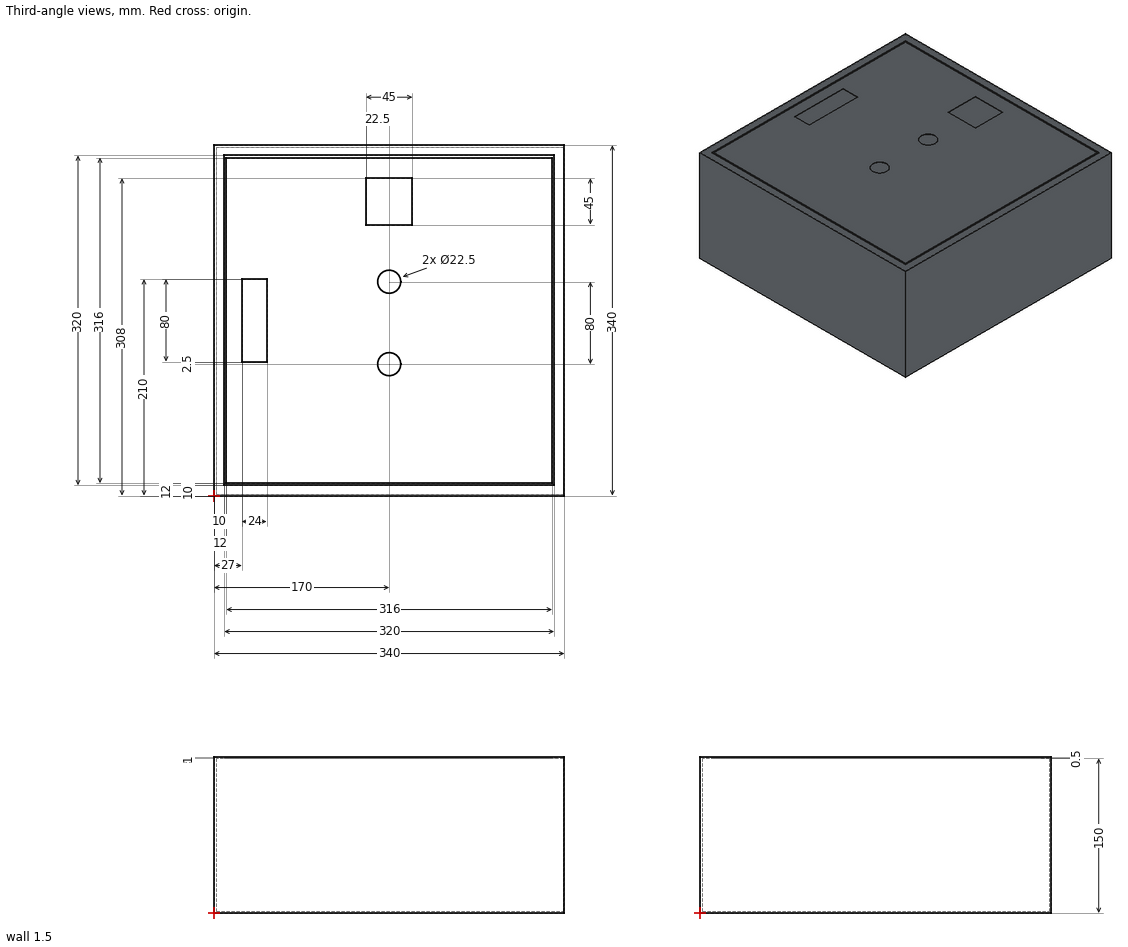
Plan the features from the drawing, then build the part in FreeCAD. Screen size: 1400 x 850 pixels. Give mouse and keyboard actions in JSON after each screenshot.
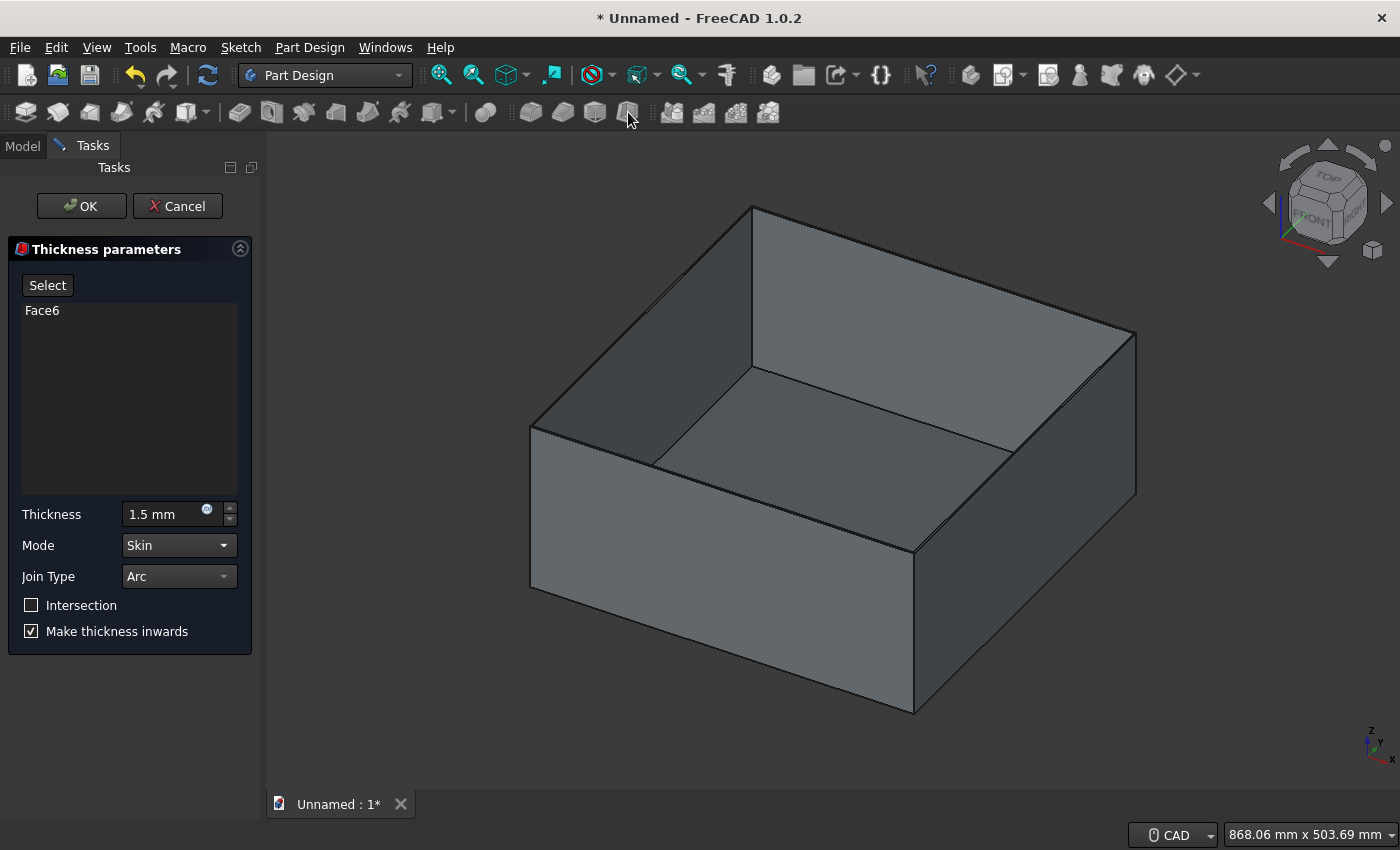
{"action": "left_click", "coordinate": [180, 576]}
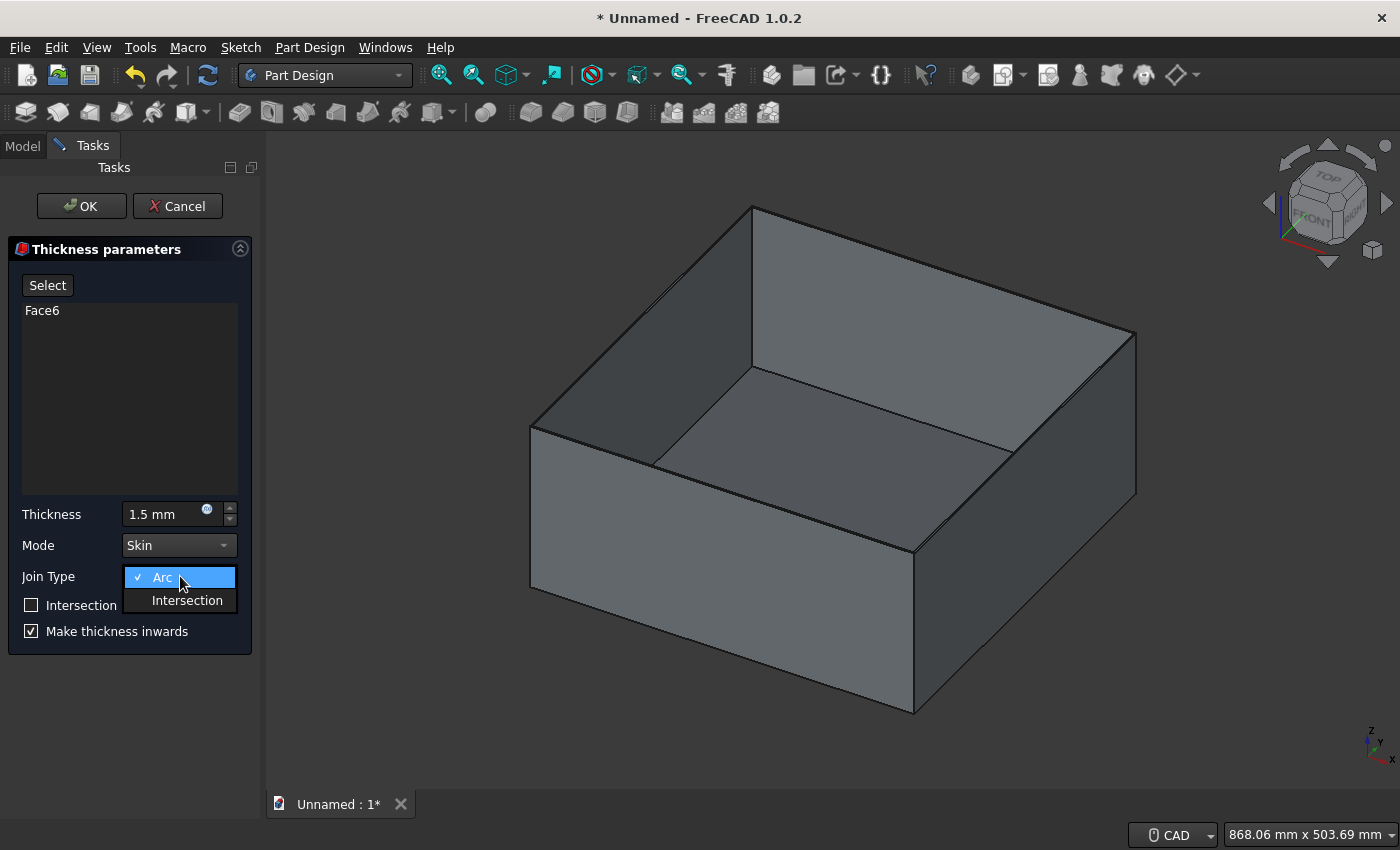
{"action": "left_click", "coordinate": [179, 600]}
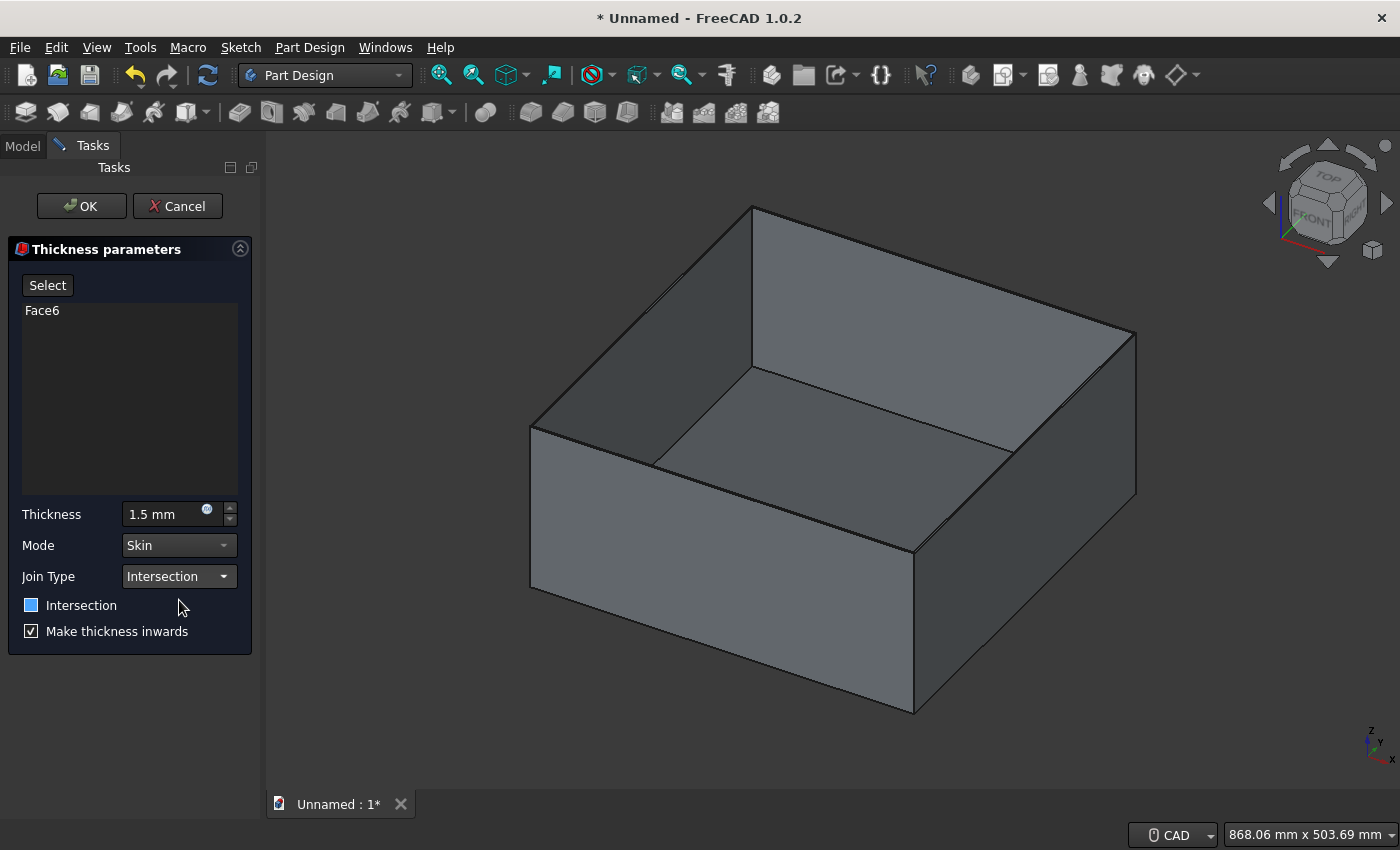
{"action": "left_click", "coordinate": [82, 206]}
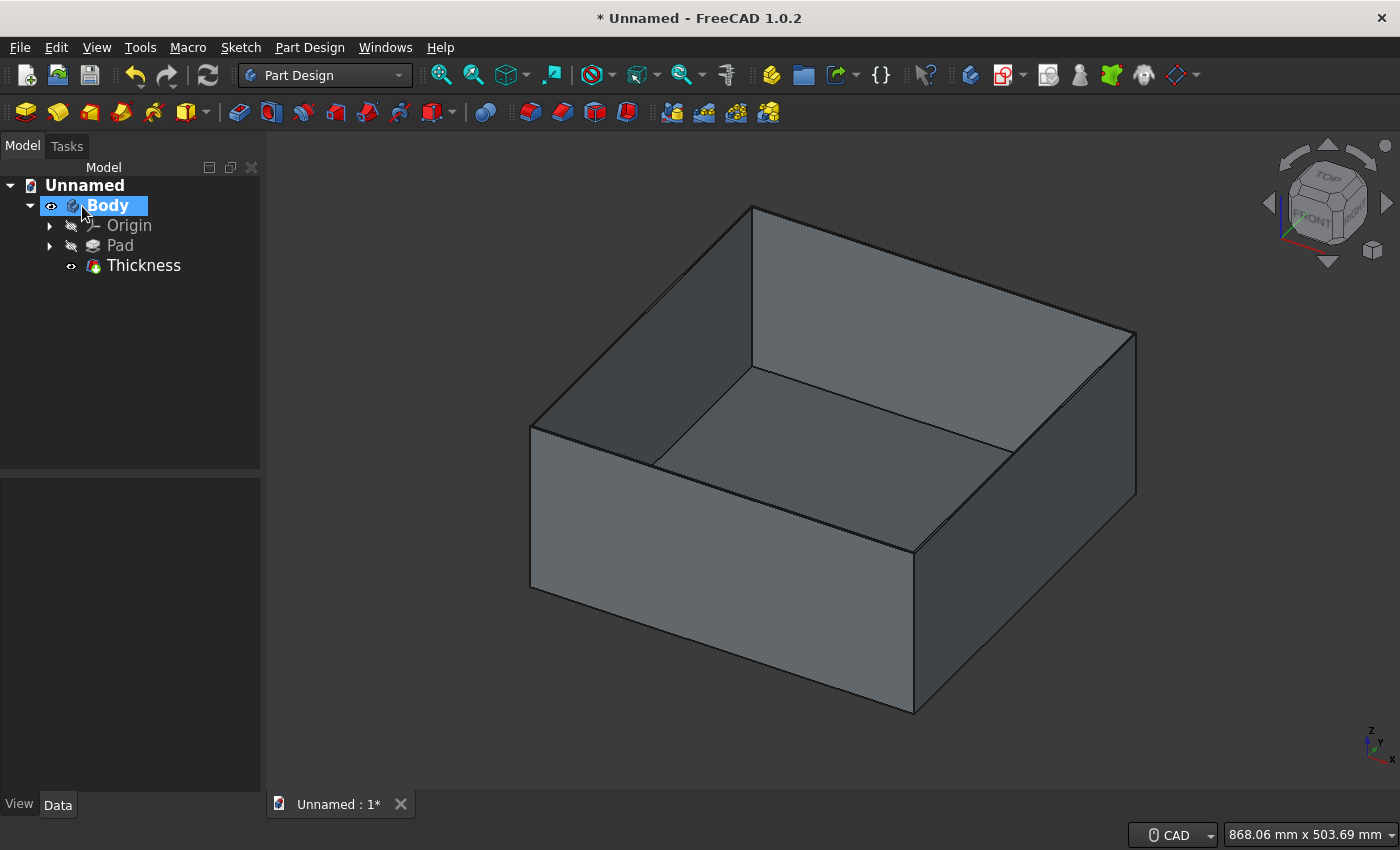
{"action": "scroll", "coordinate": [988, 479], "scroll_direction": "up", "scroll_amount": 15}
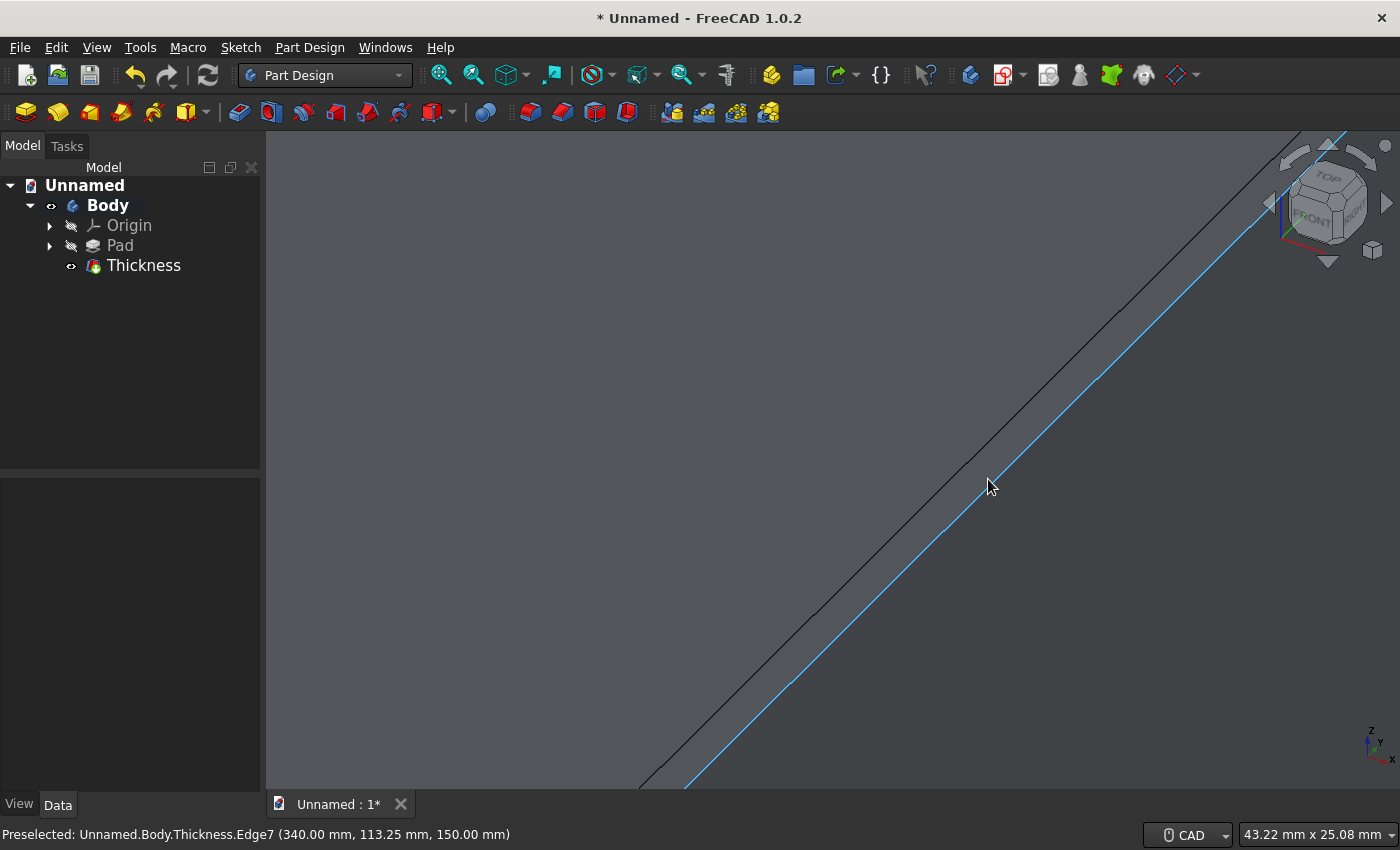
{"action": "left_click", "coordinate": [977, 482]}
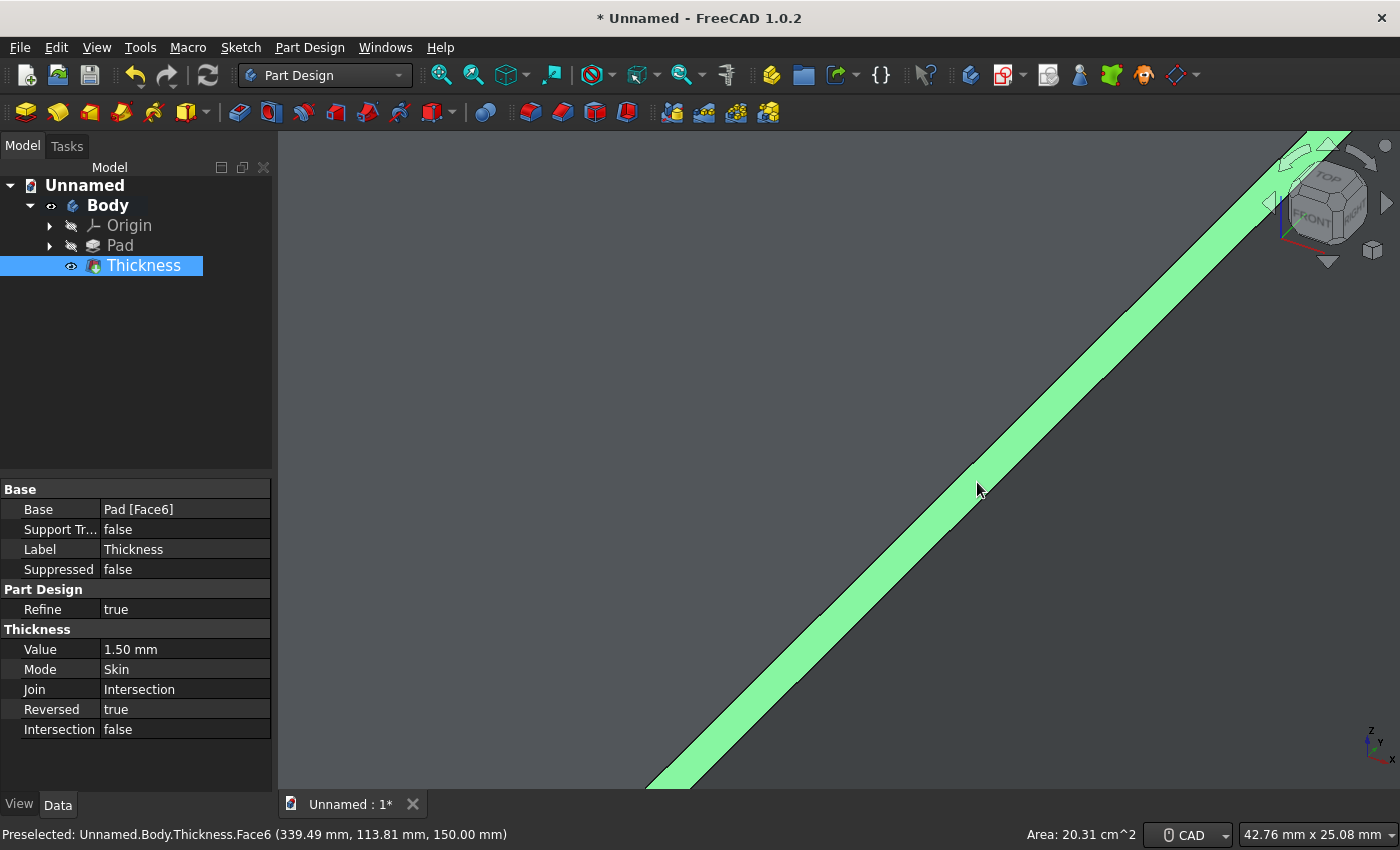
{"action": "left_click", "coordinate": [1004, 76]}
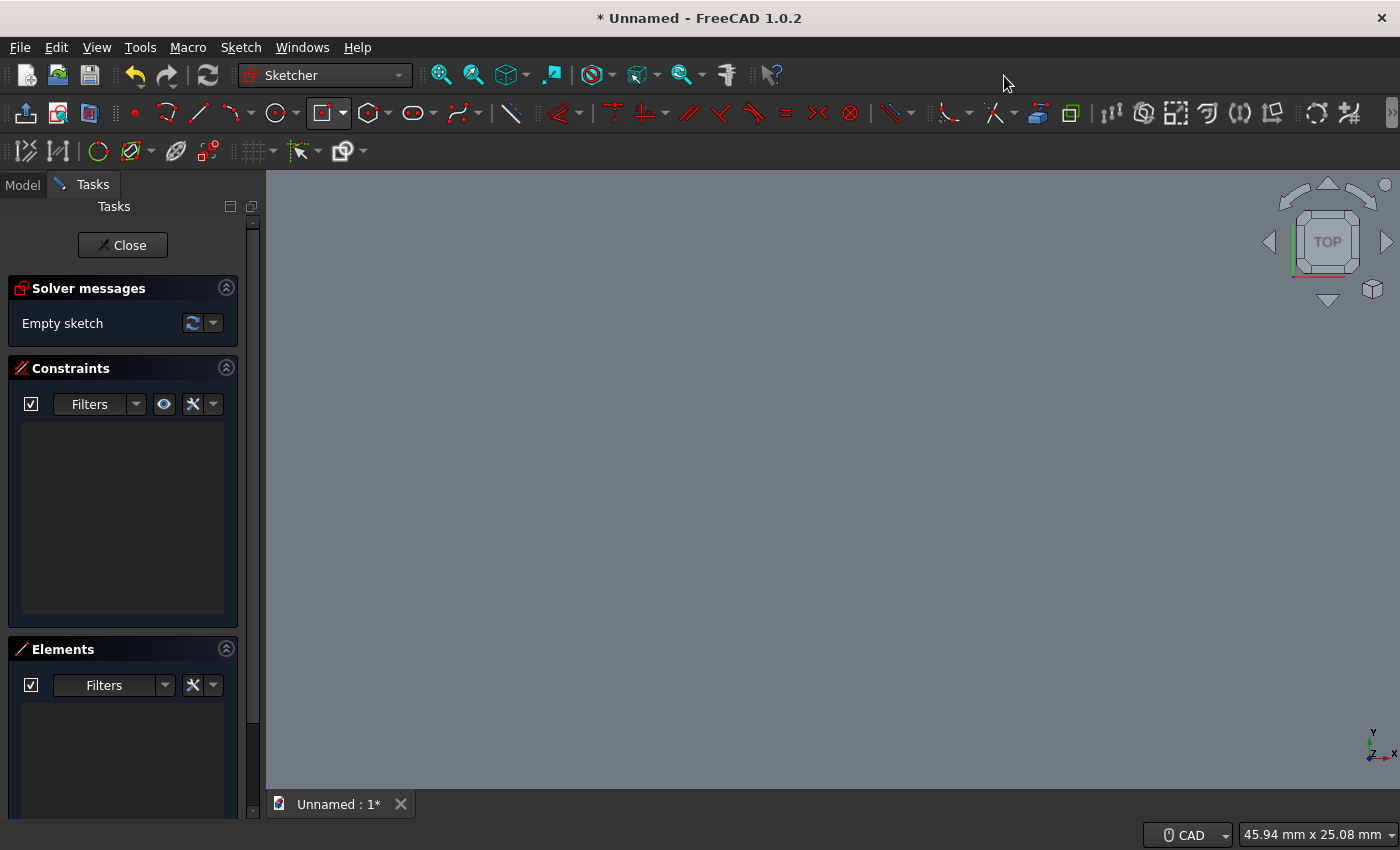
{"action": "scroll", "coordinate": [893, 415], "scroll_direction": "down", "scroll_amount": 15}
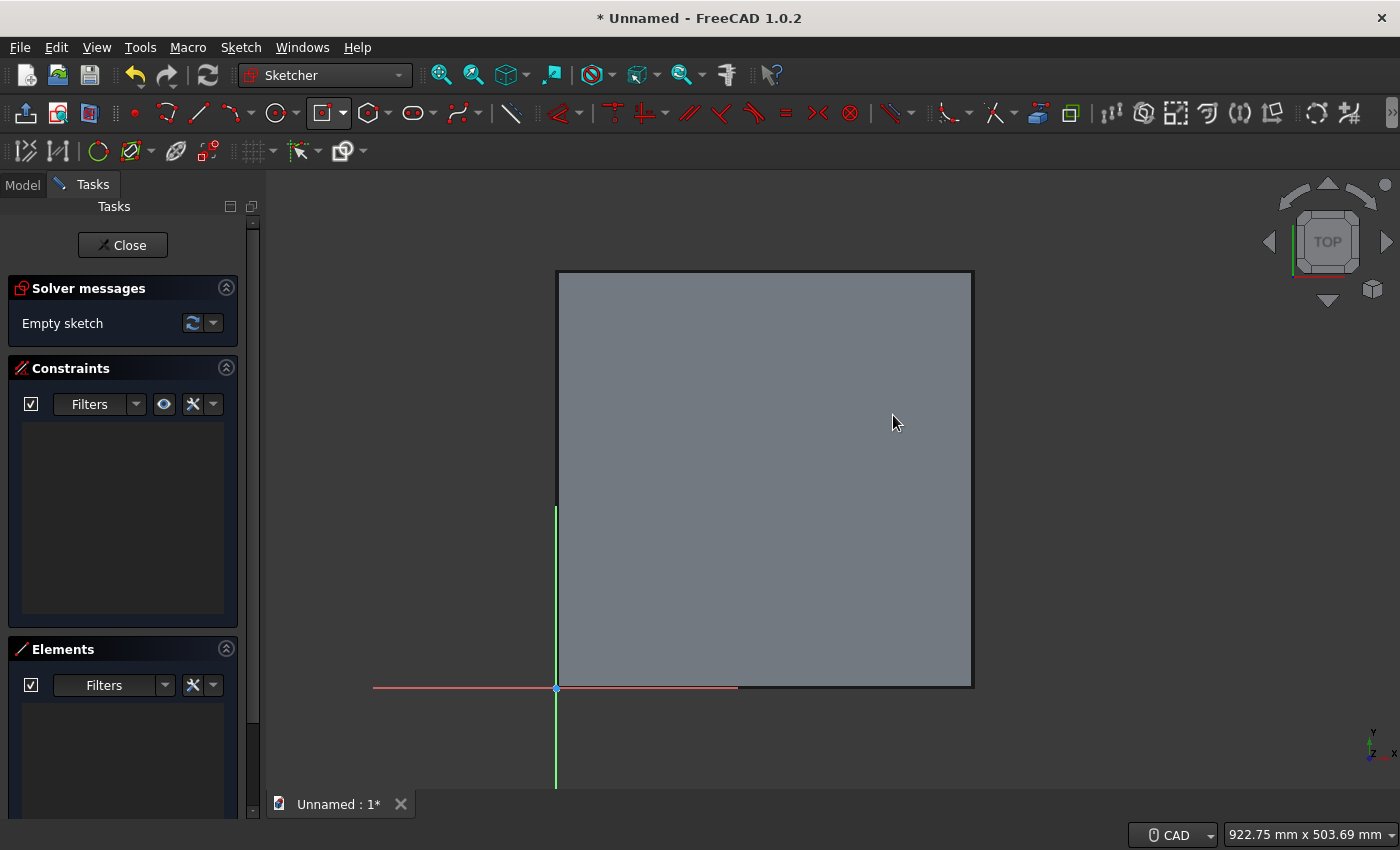
{"action": "key", "text": "g r"}